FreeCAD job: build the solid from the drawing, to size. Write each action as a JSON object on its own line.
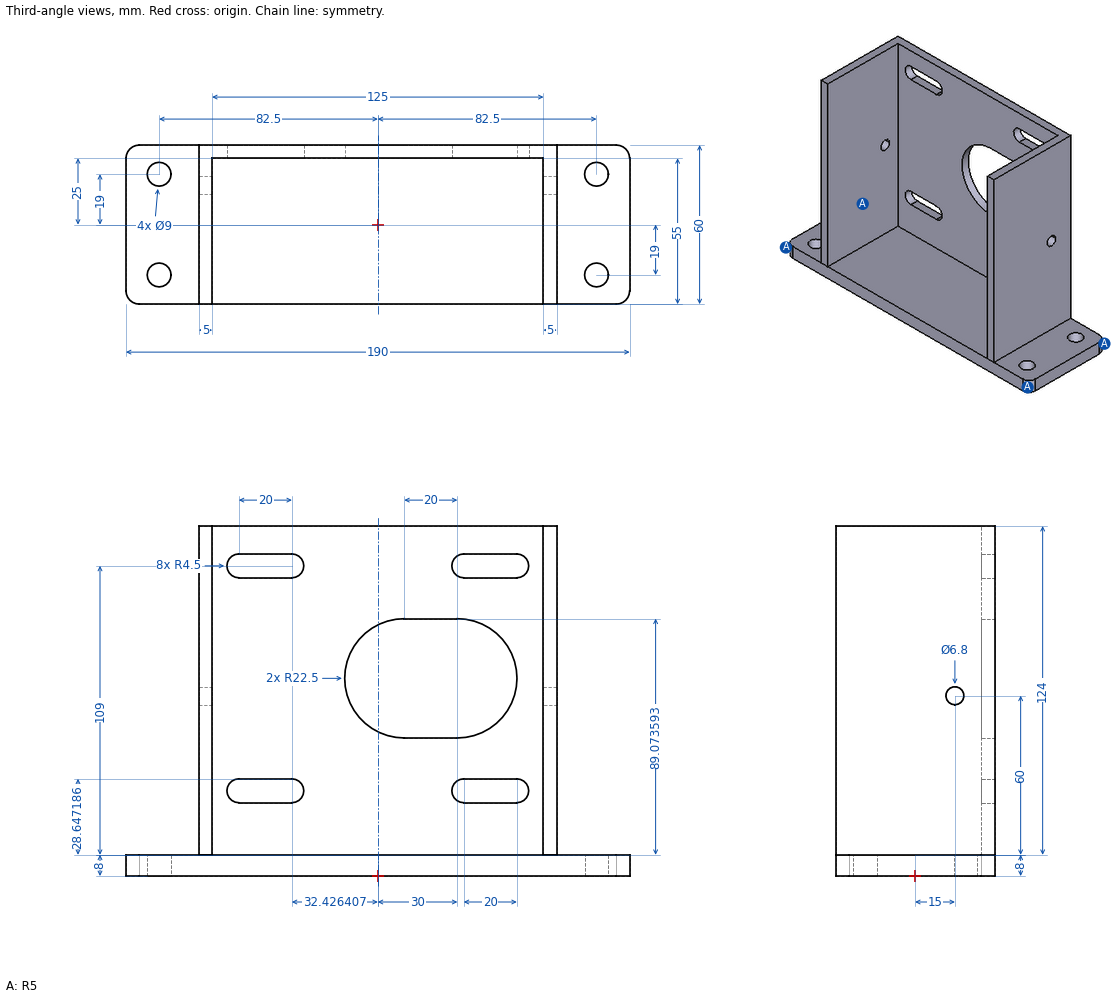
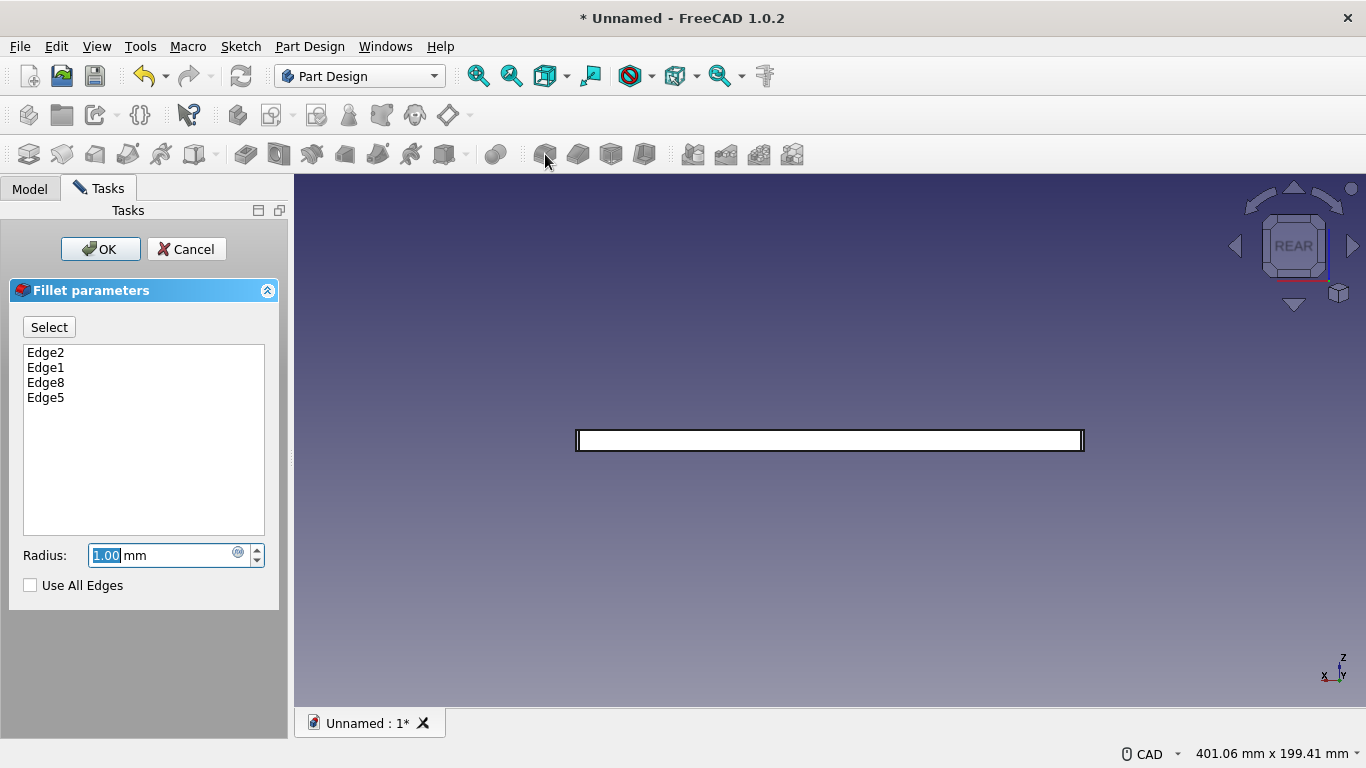
{"action": "type", "text": "5"}
{"action": "key", "text": "Tab"}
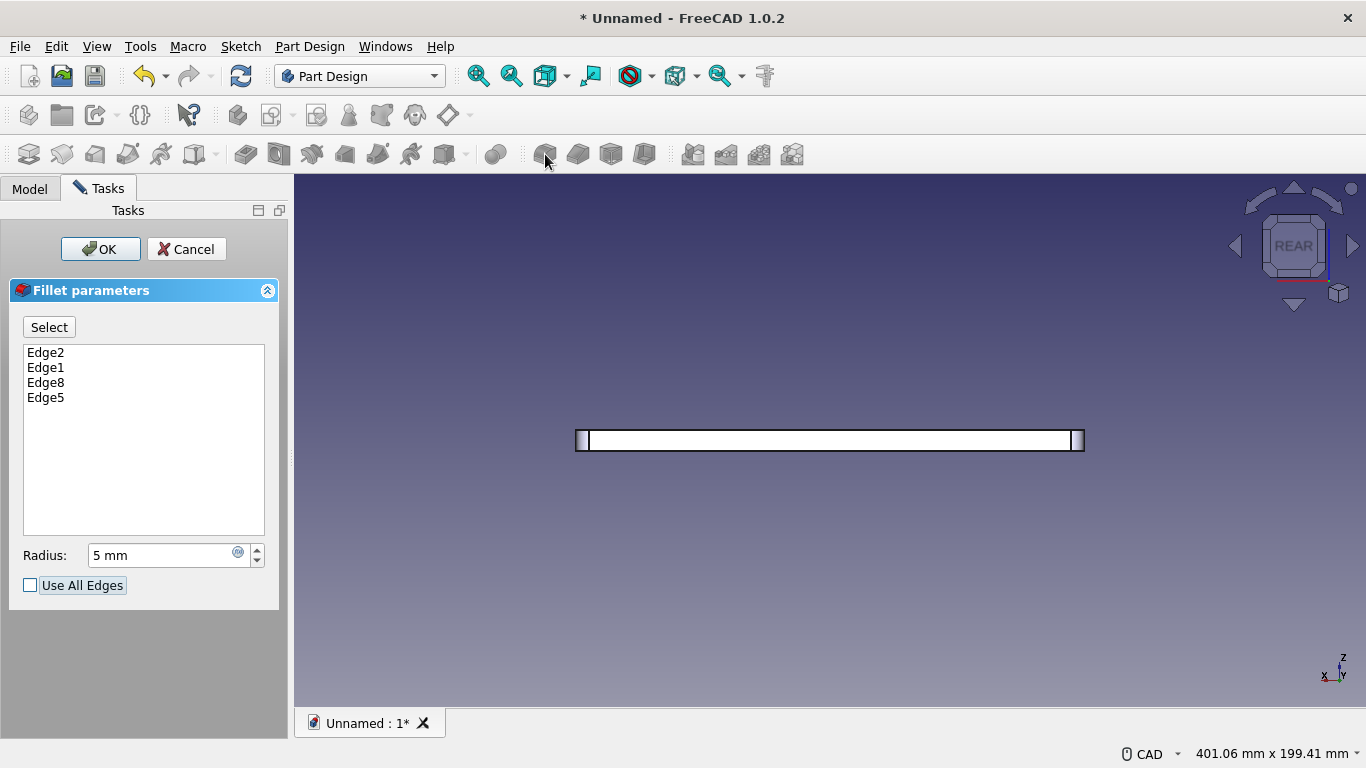
{"action": "left_click", "coordinate": [101, 249]}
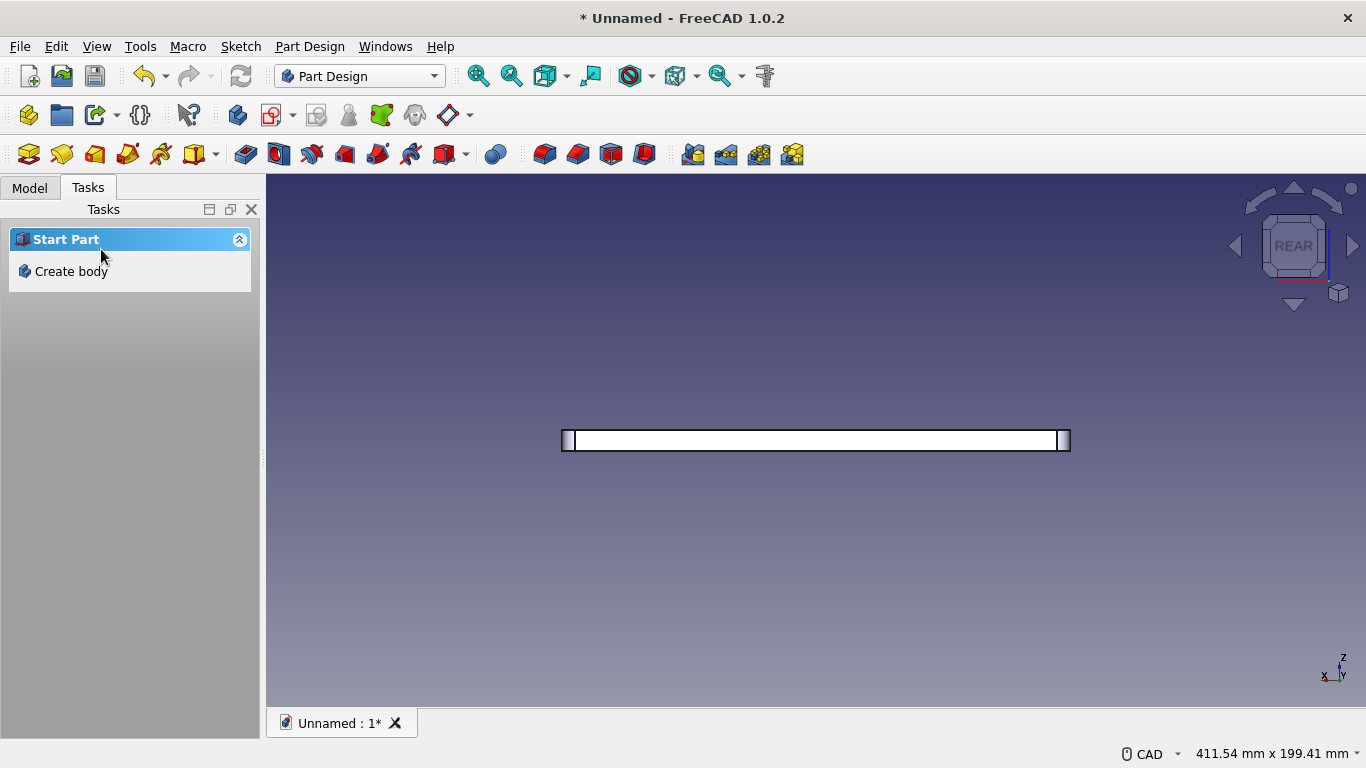
{"action": "left_click", "coordinate": [238, 116]}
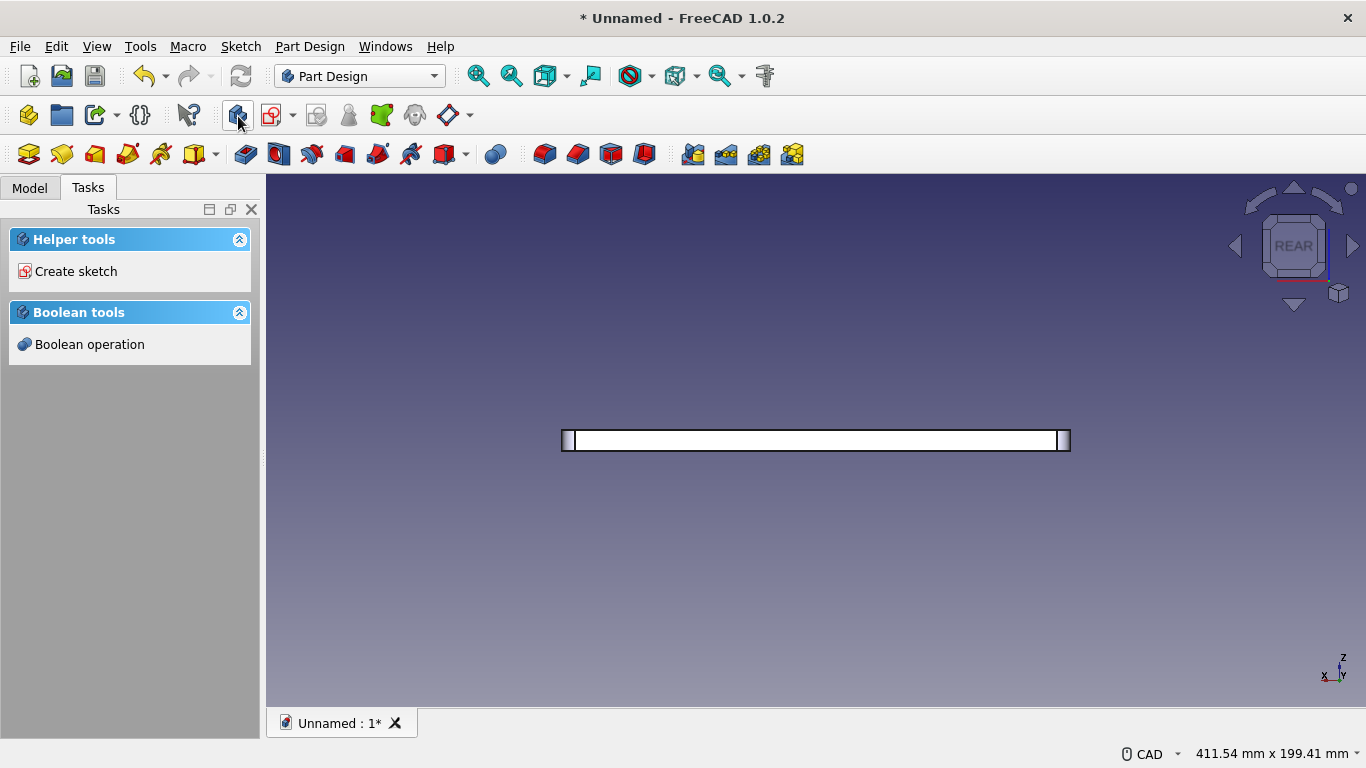
{"action": "left_click", "coordinate": [30, 188]}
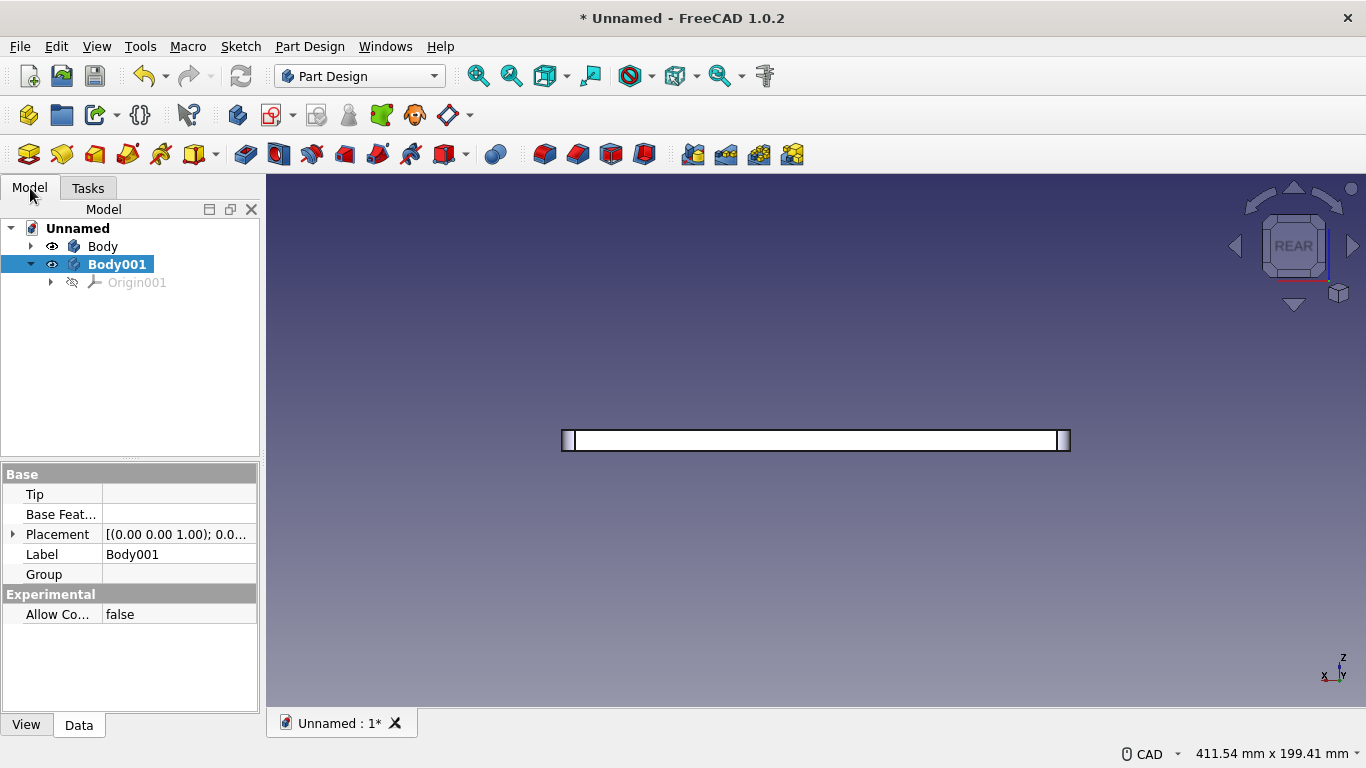
{"action": "left_click", "coordinate": [51, 282]}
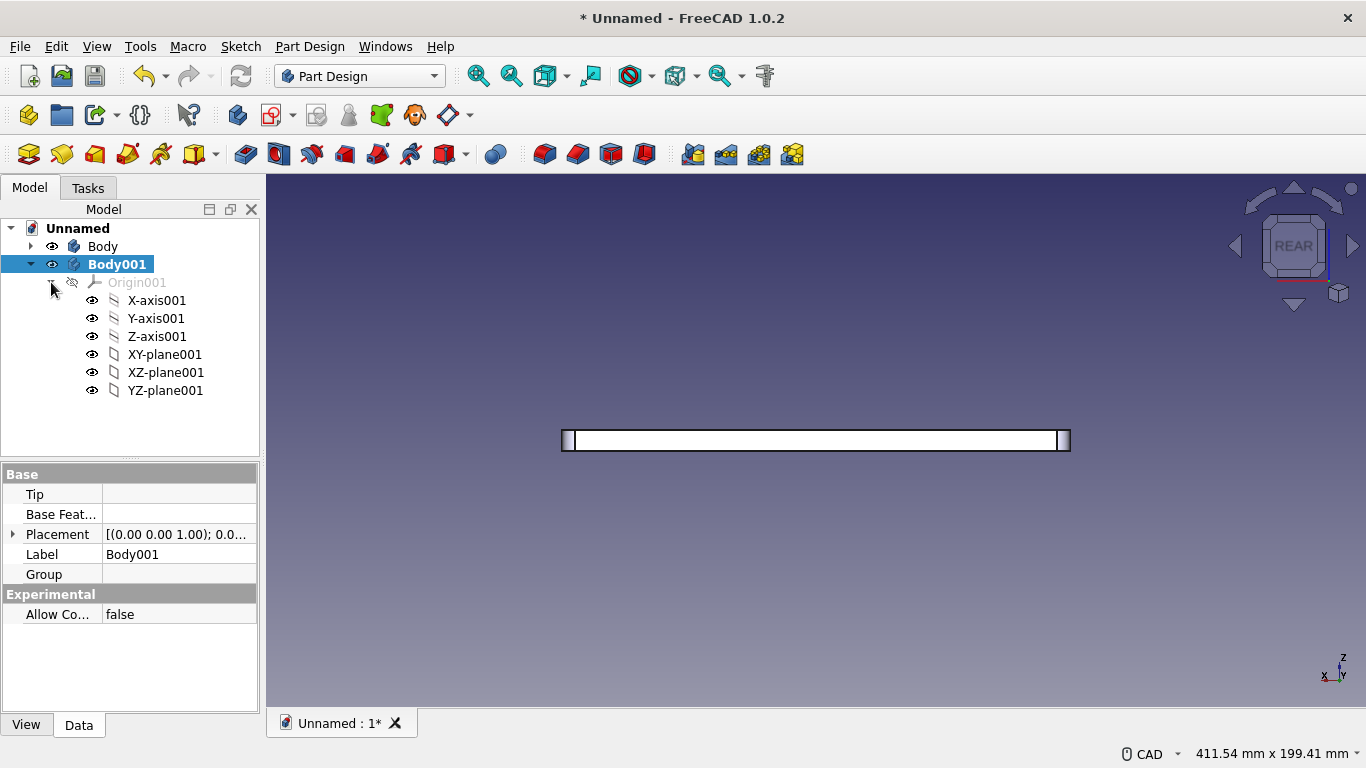
{"action": "left_click", "coordinate": [137, 354]}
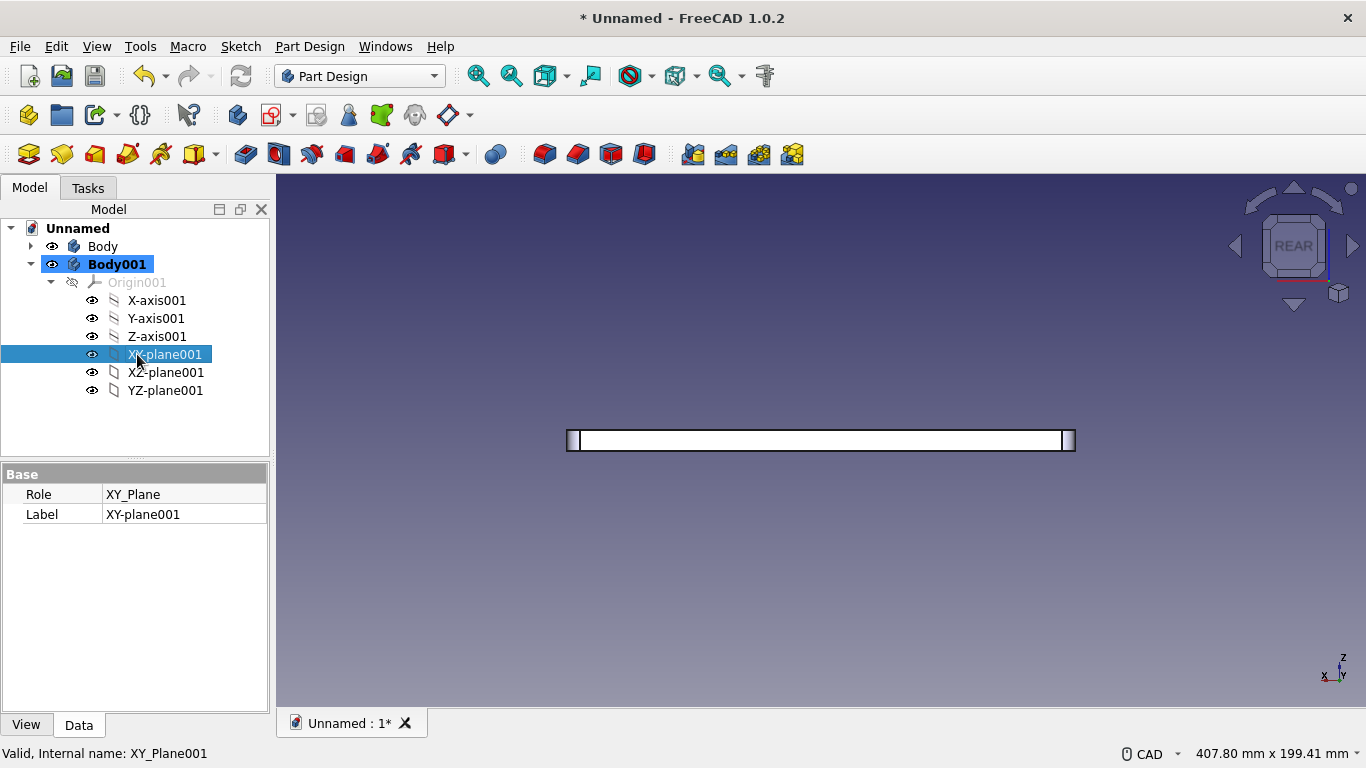
{"action": "left_click", "coordinate": [448, 116]}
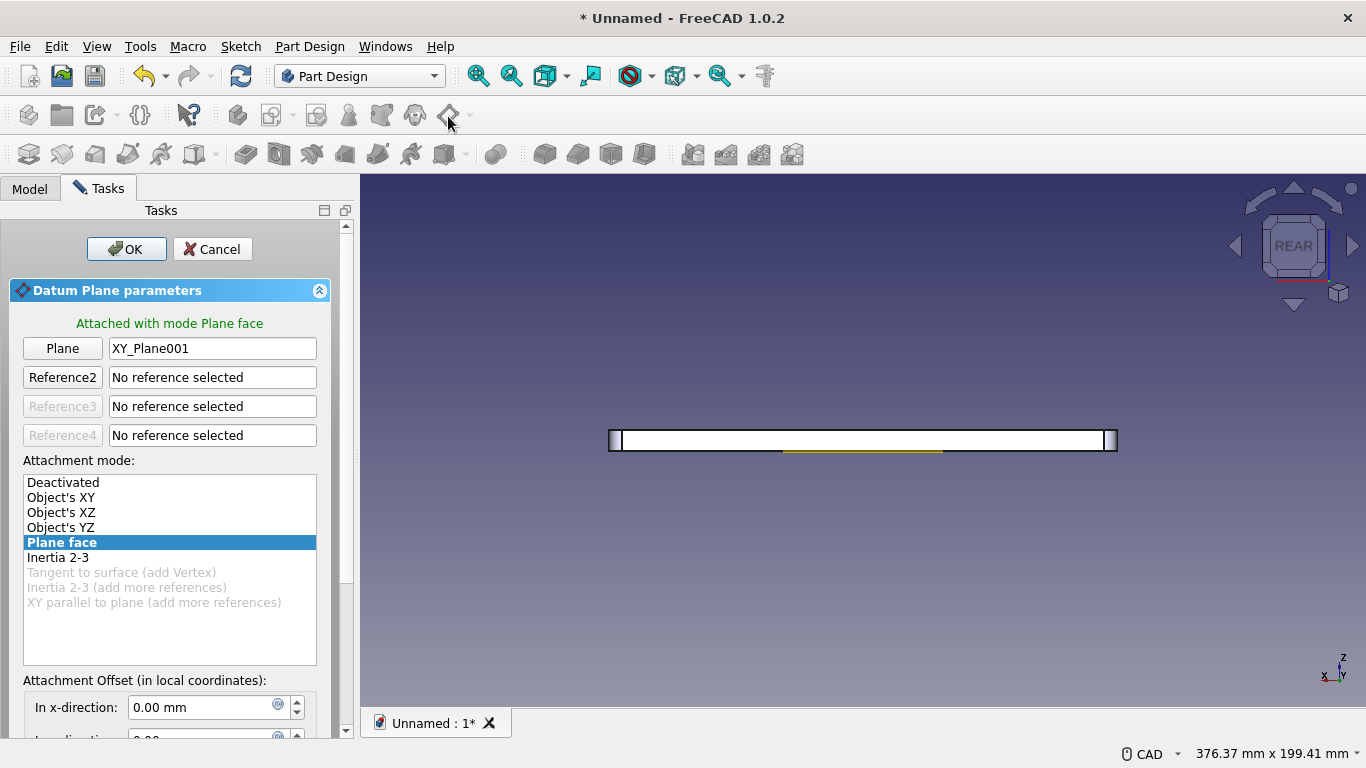
{"action": "scroll", "coordinate": [346, 479], "scroll_direction": "down", "scroll_amount": 2}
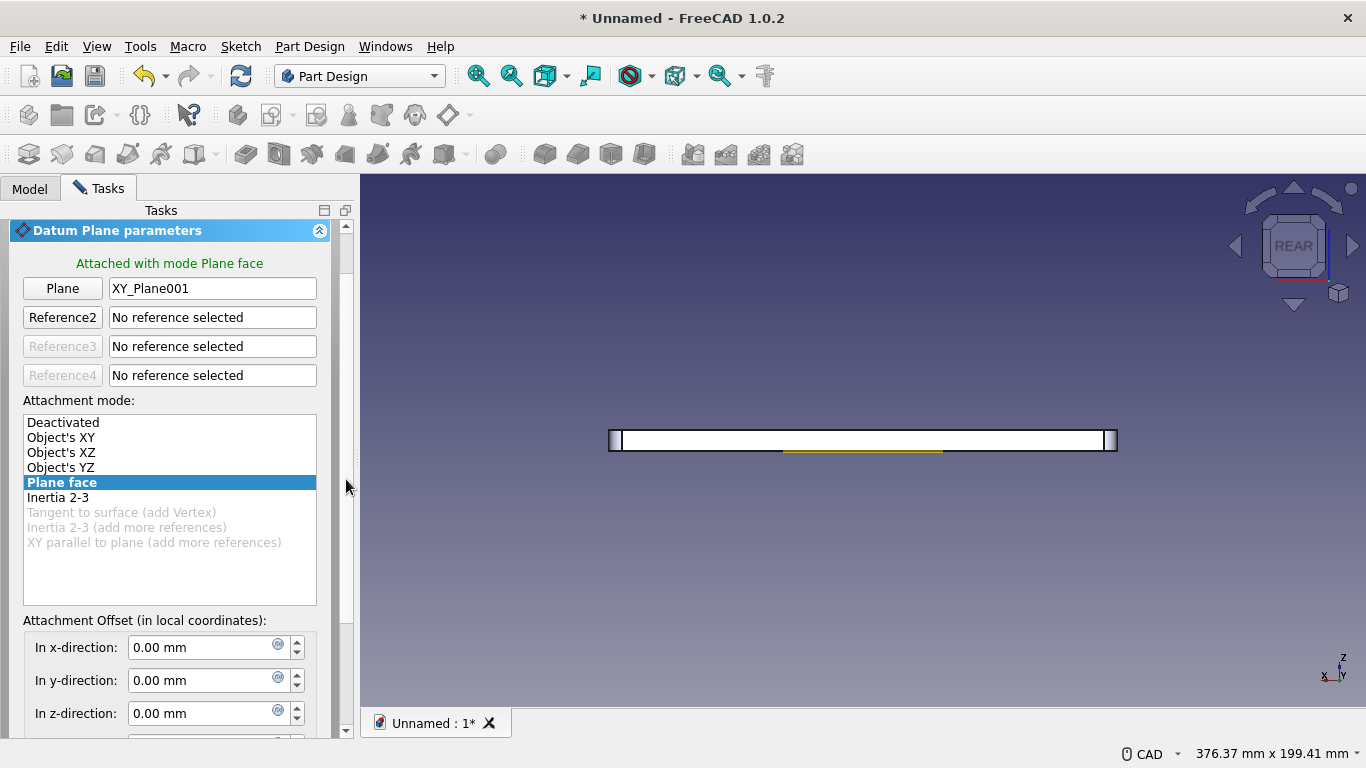
{"action": "triple_click", "coordinate": [210, 654]}